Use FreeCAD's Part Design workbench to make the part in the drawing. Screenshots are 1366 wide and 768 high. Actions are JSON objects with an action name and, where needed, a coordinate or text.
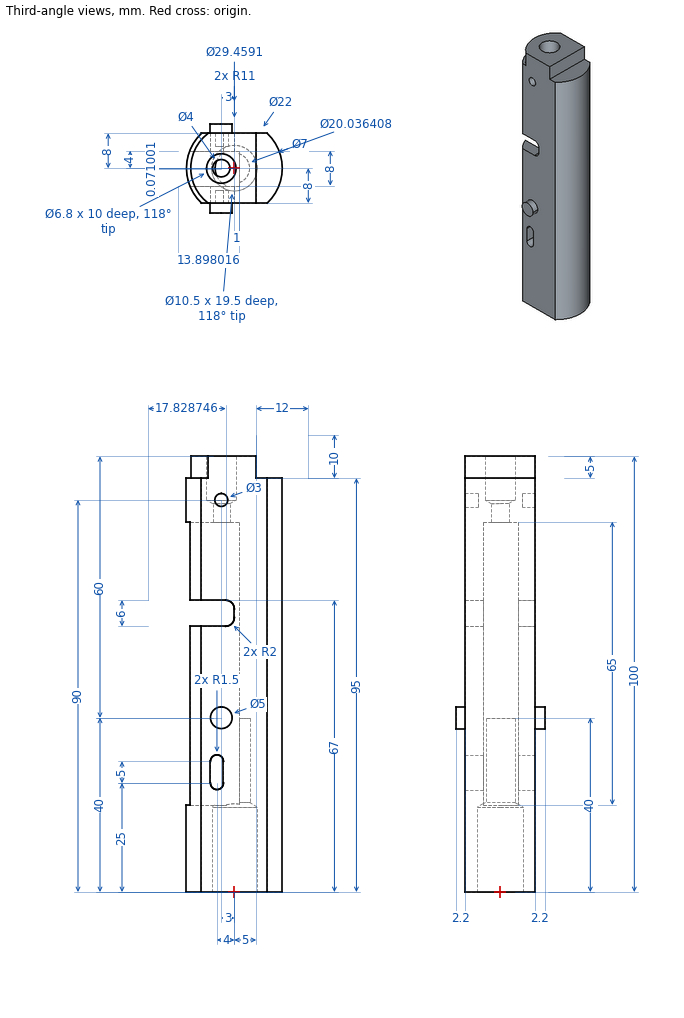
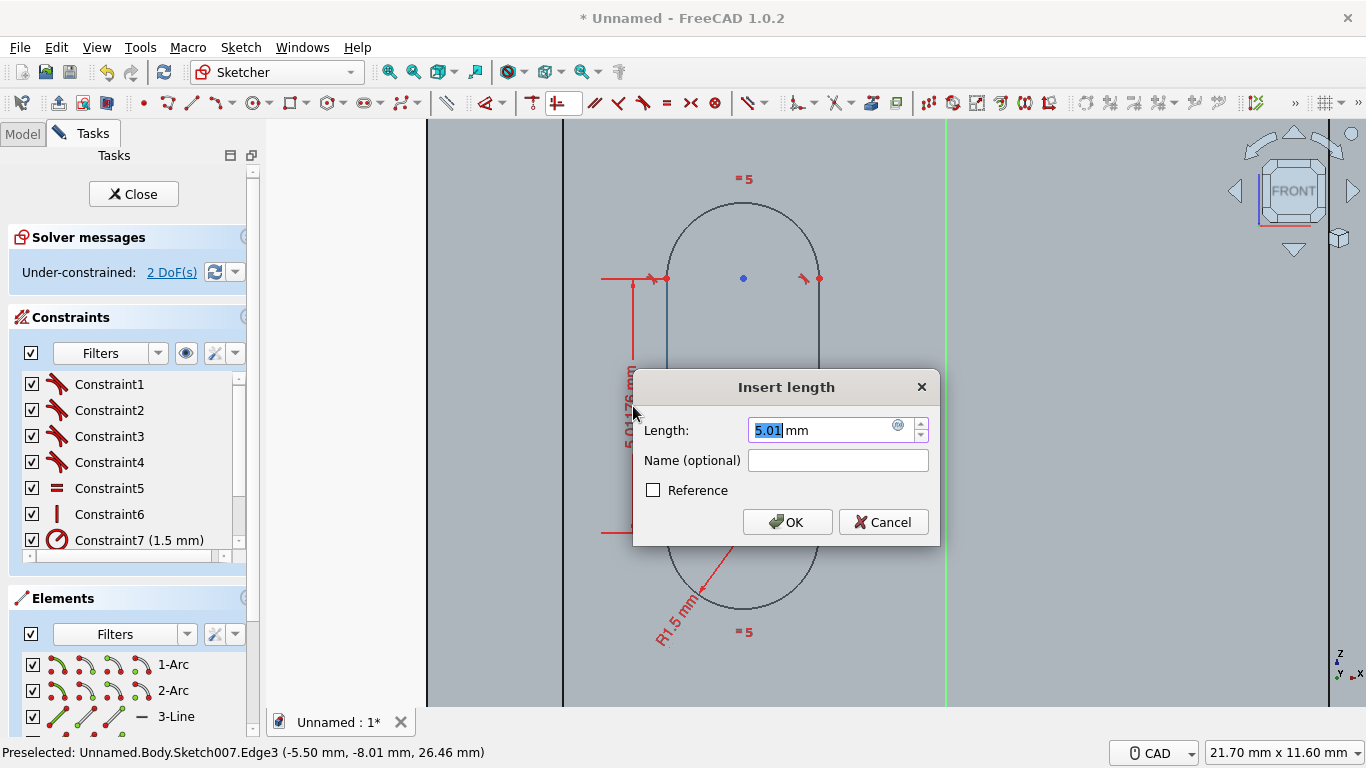
{"action": "type", "text": "5"}
{"action": "key", "text": "Return"}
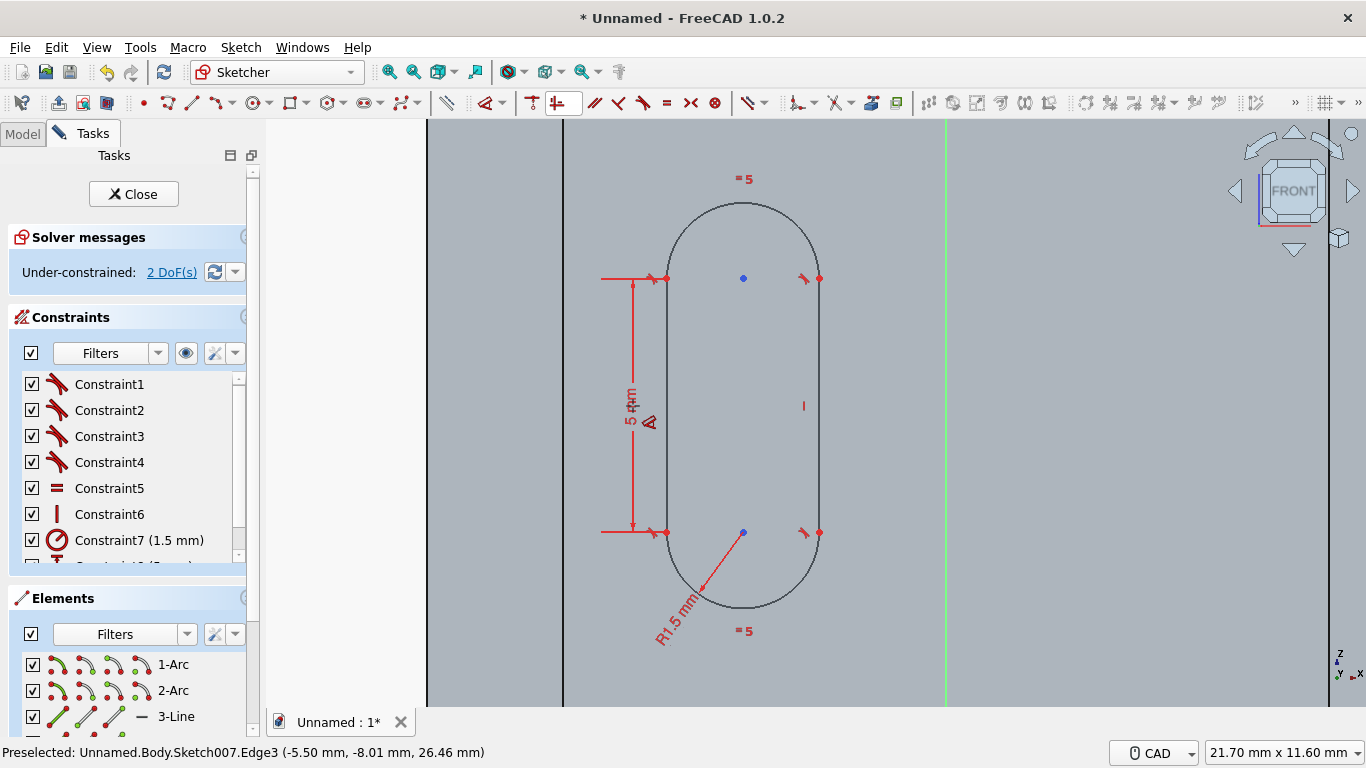
{"action": "left_click", "coordinate": [743, 532]}
{"action": "left_click", "coordinate": [844, 498]}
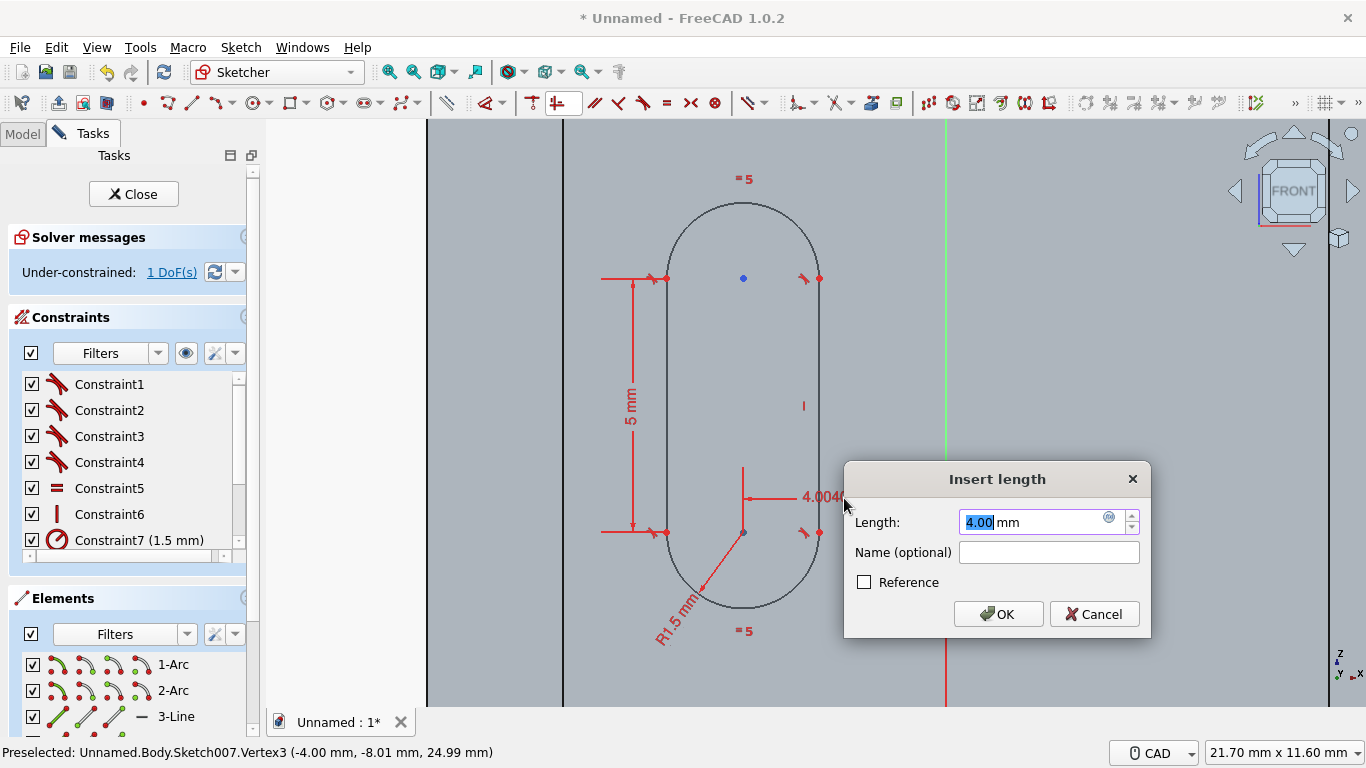
{"action": "type", "text": "4"}
{"action": "key", "text": "Return"}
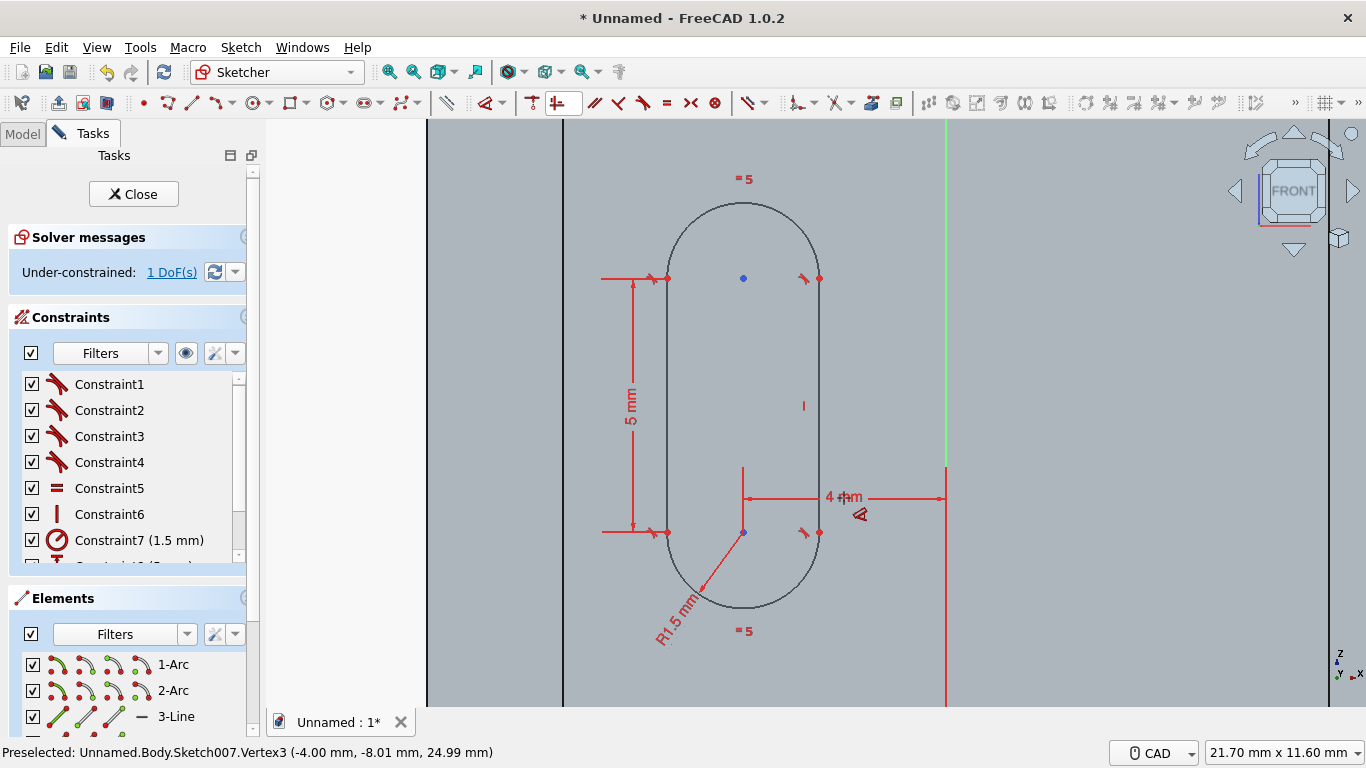
{"action": "left_click", "coordinate": [667, 532]}
{"action": "left_click", "coordinate": [980, 606]}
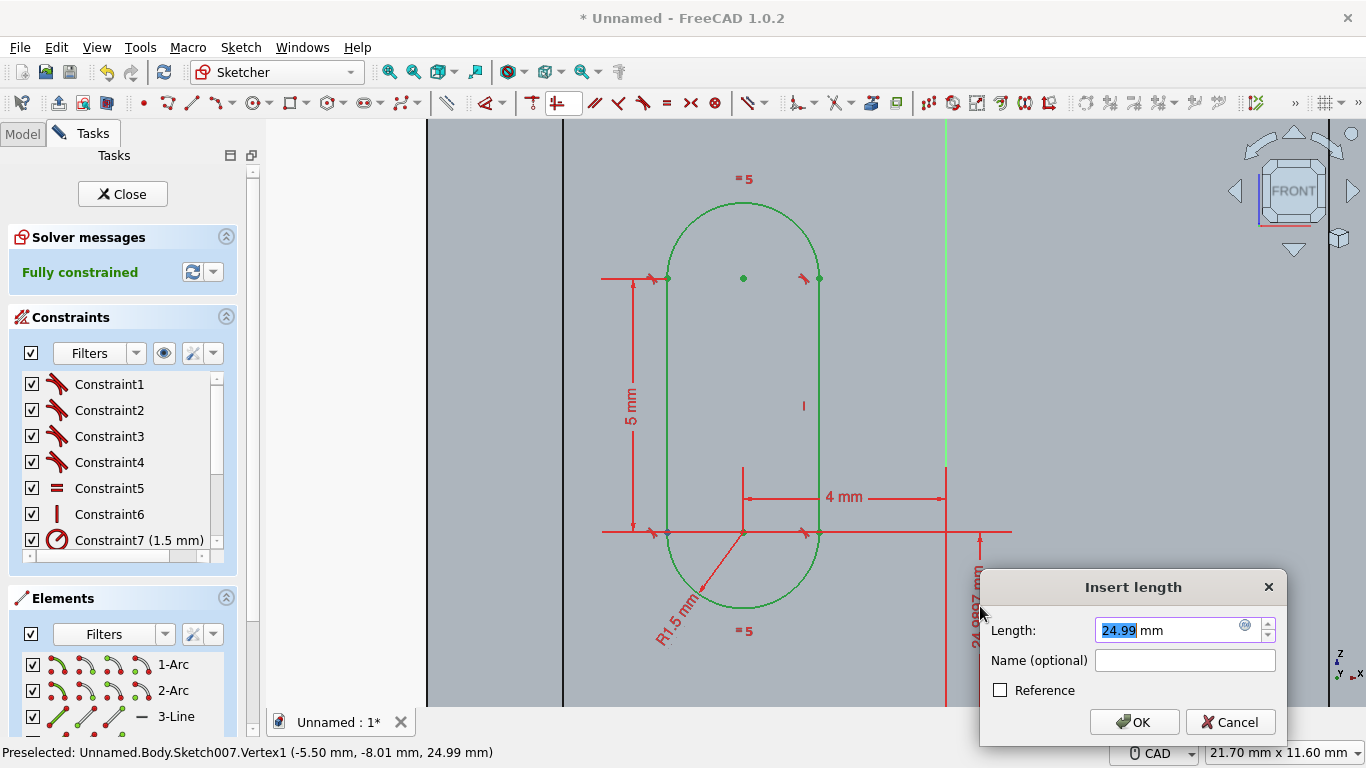
{"action": "type", "text": "25"}
{"action": "key", "text": "Return"}
{"action": "key", "text": "Escape"}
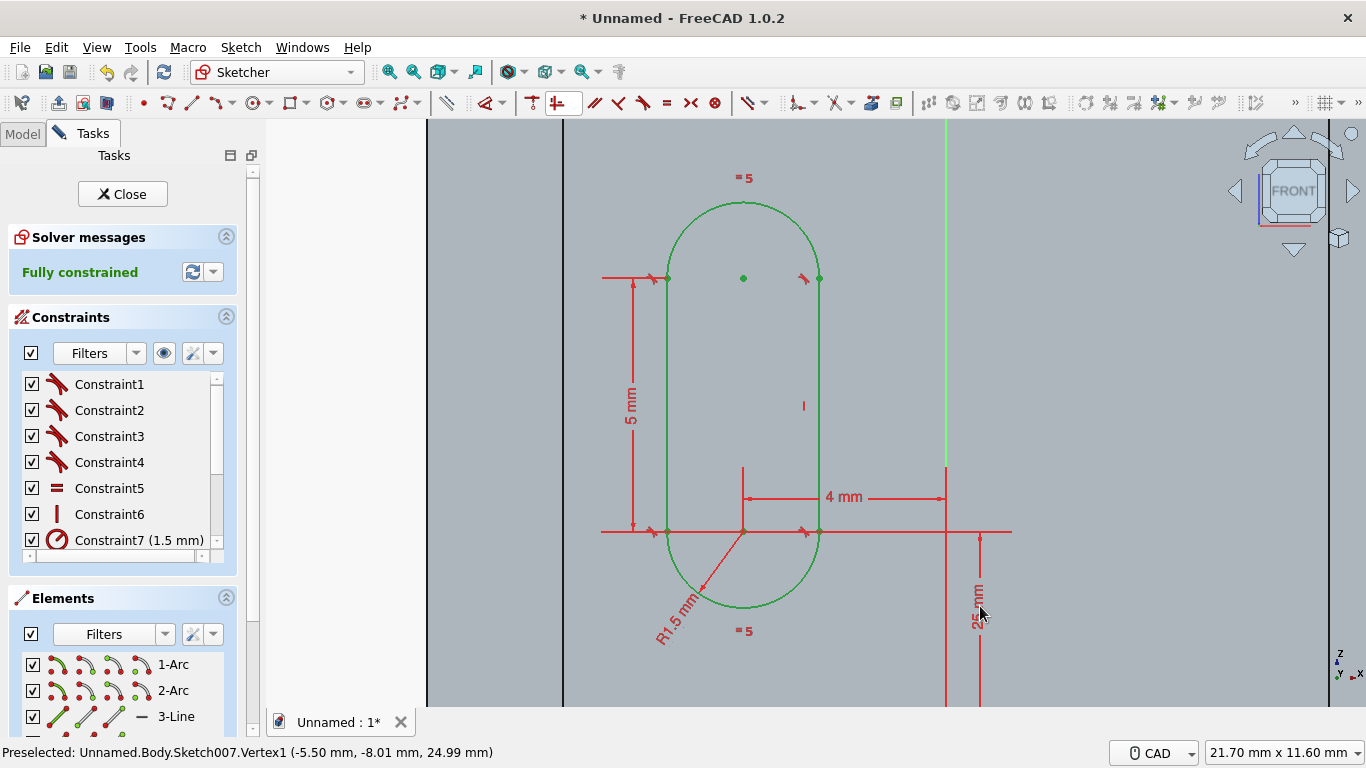
{"action": "left_click", "coordinate": [123, 194]}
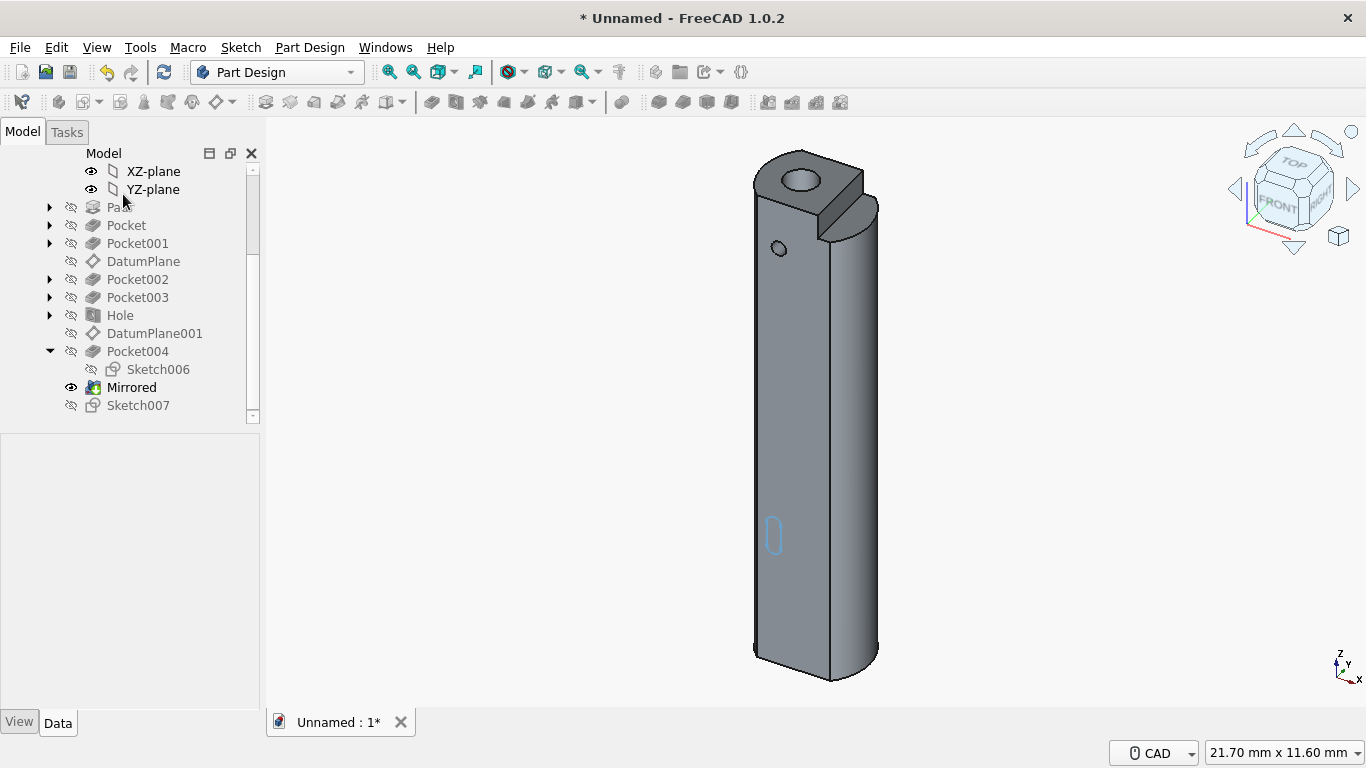
{"action": "left_click", "coordinate": [432, 102]}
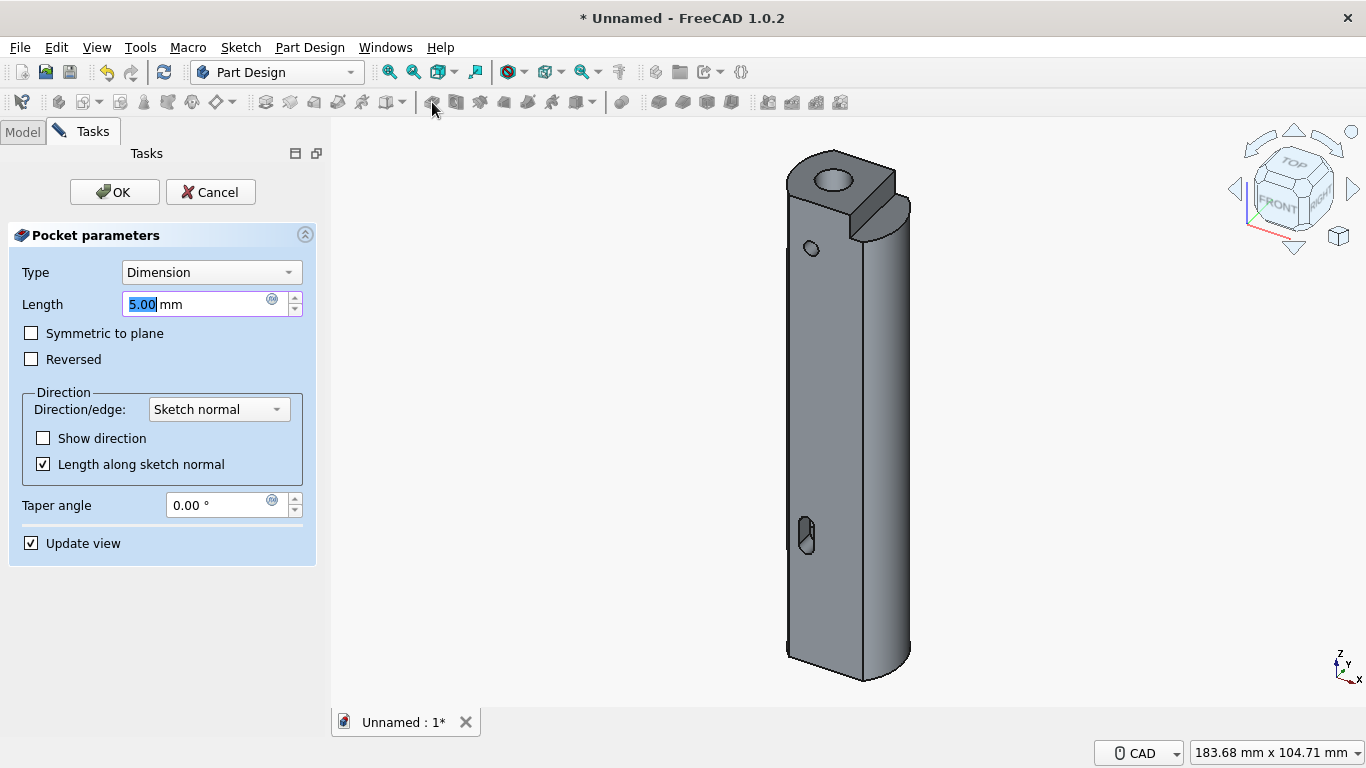
{"action": "left_click", "coordinate": [212, 272]}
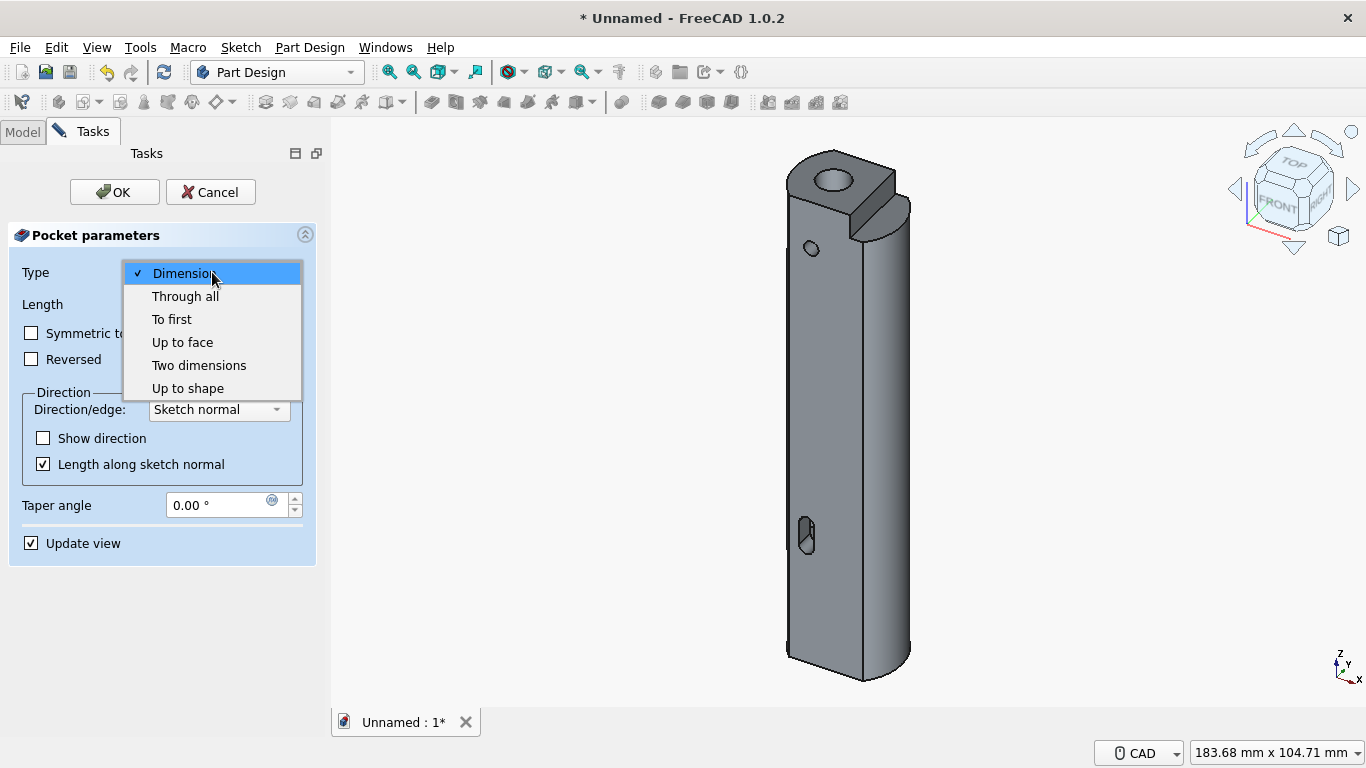
{"action": "left_click", "coordinate": [212, 296]}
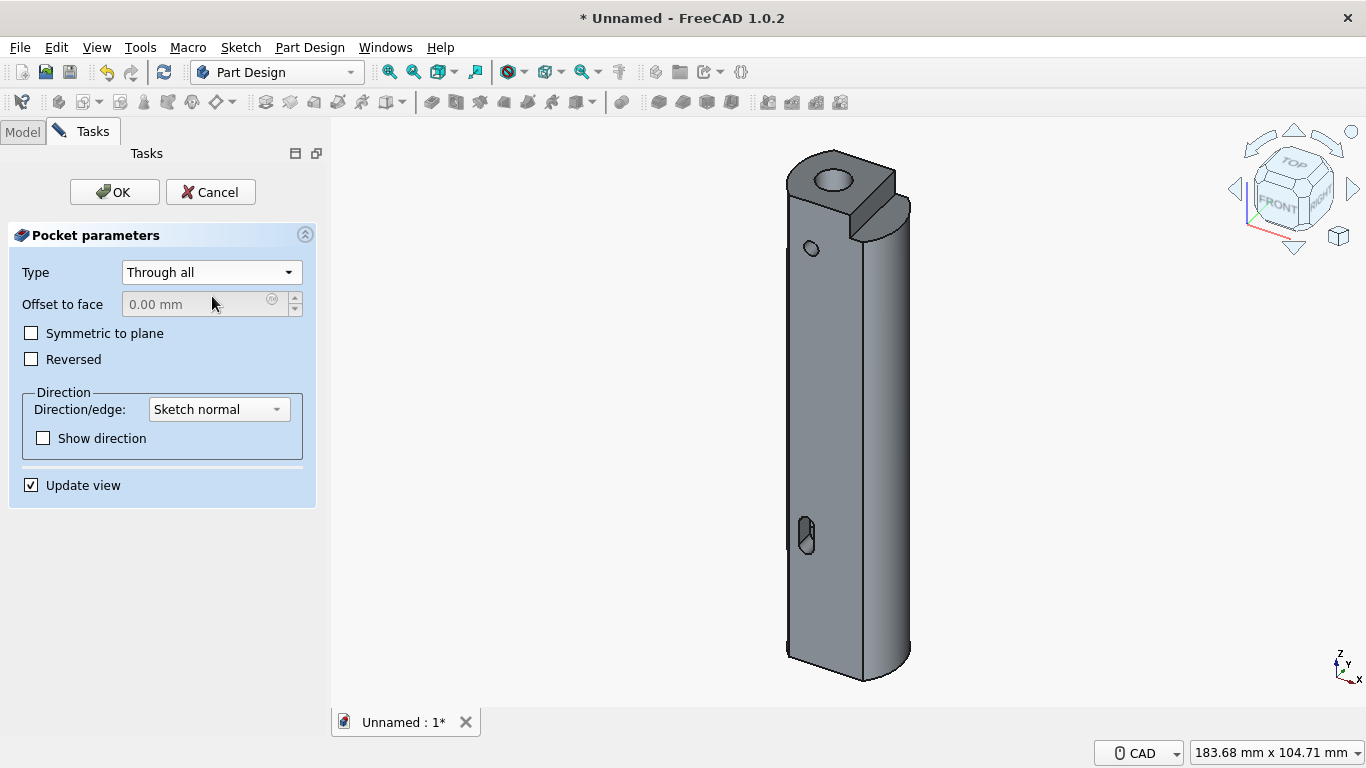
{"action": "left_click", "coordinate": [115, 192]}